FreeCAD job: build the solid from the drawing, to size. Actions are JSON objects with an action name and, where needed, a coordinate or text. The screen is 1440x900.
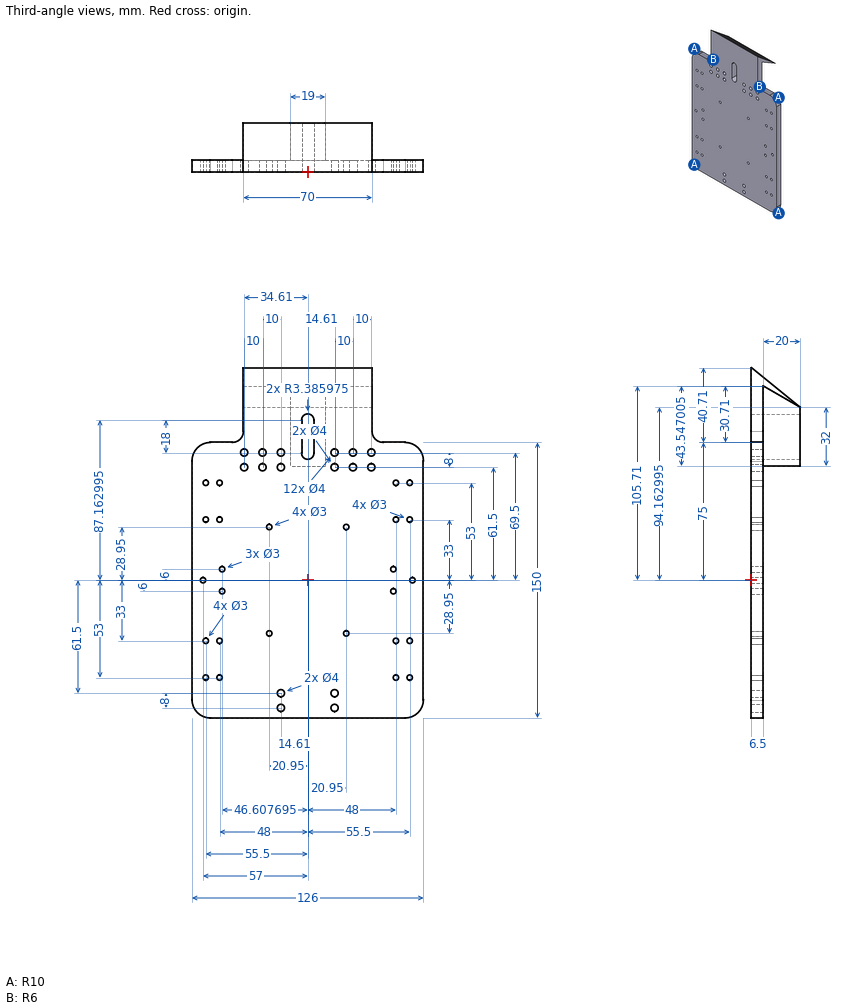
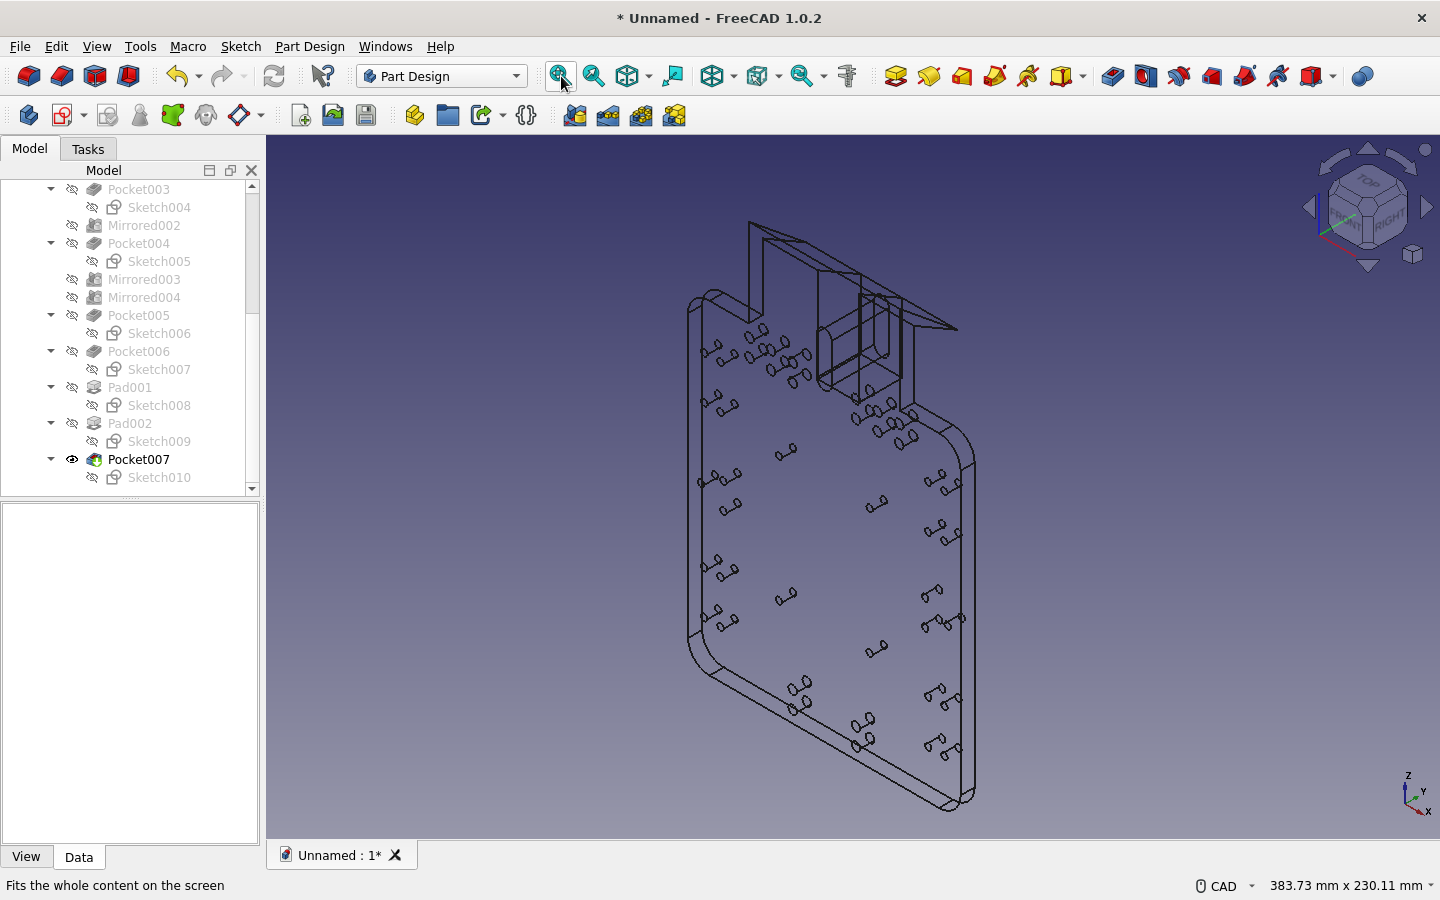
{"action": "left_click", "coordinate": [756, 318]}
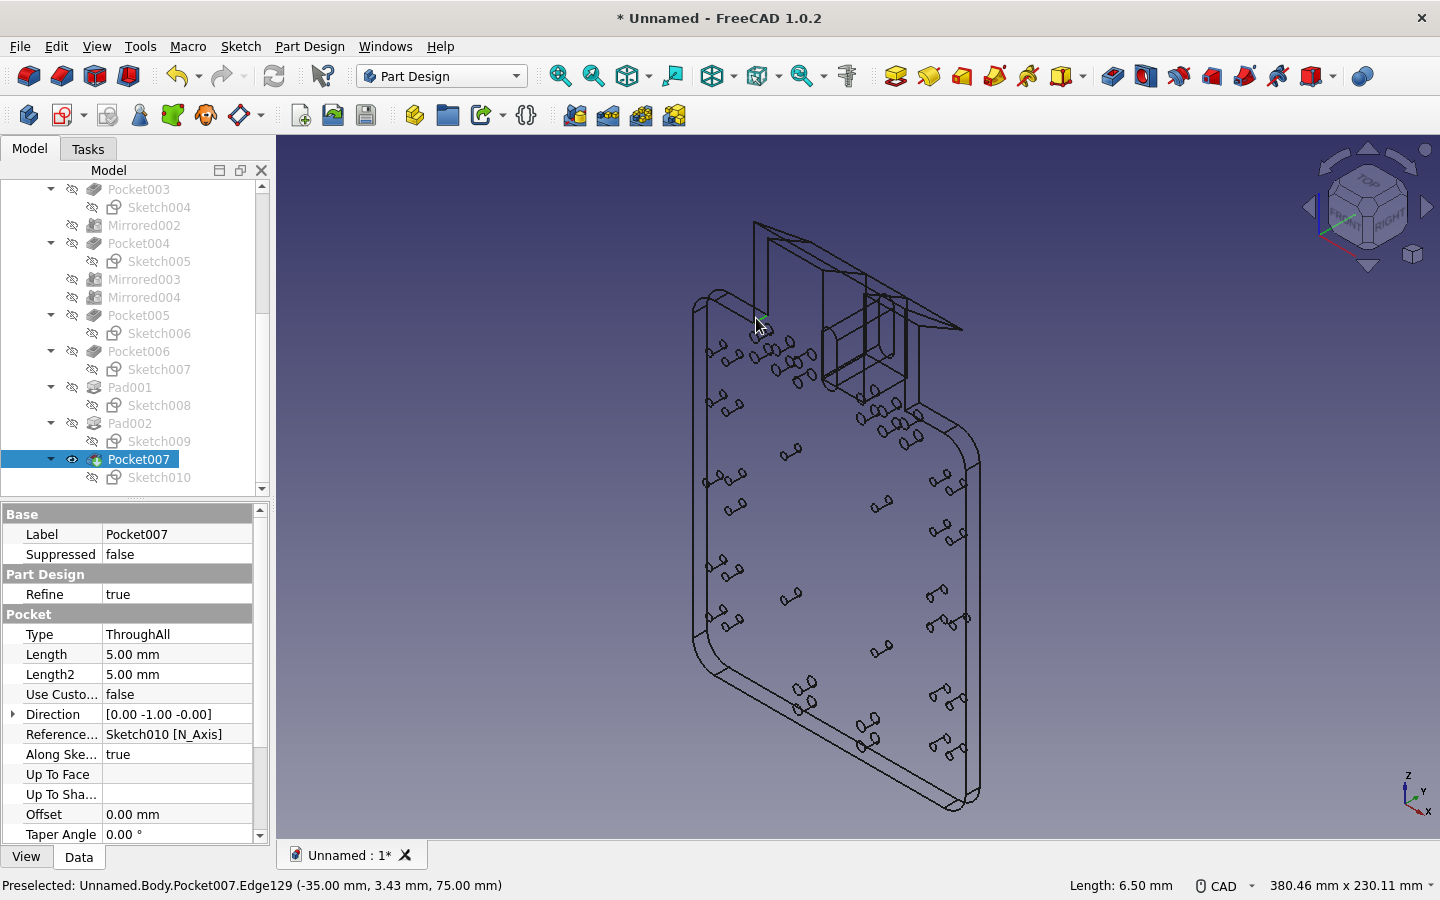
{"action": "left_click", "coordinate": [912, 406], "text": "ctrl"}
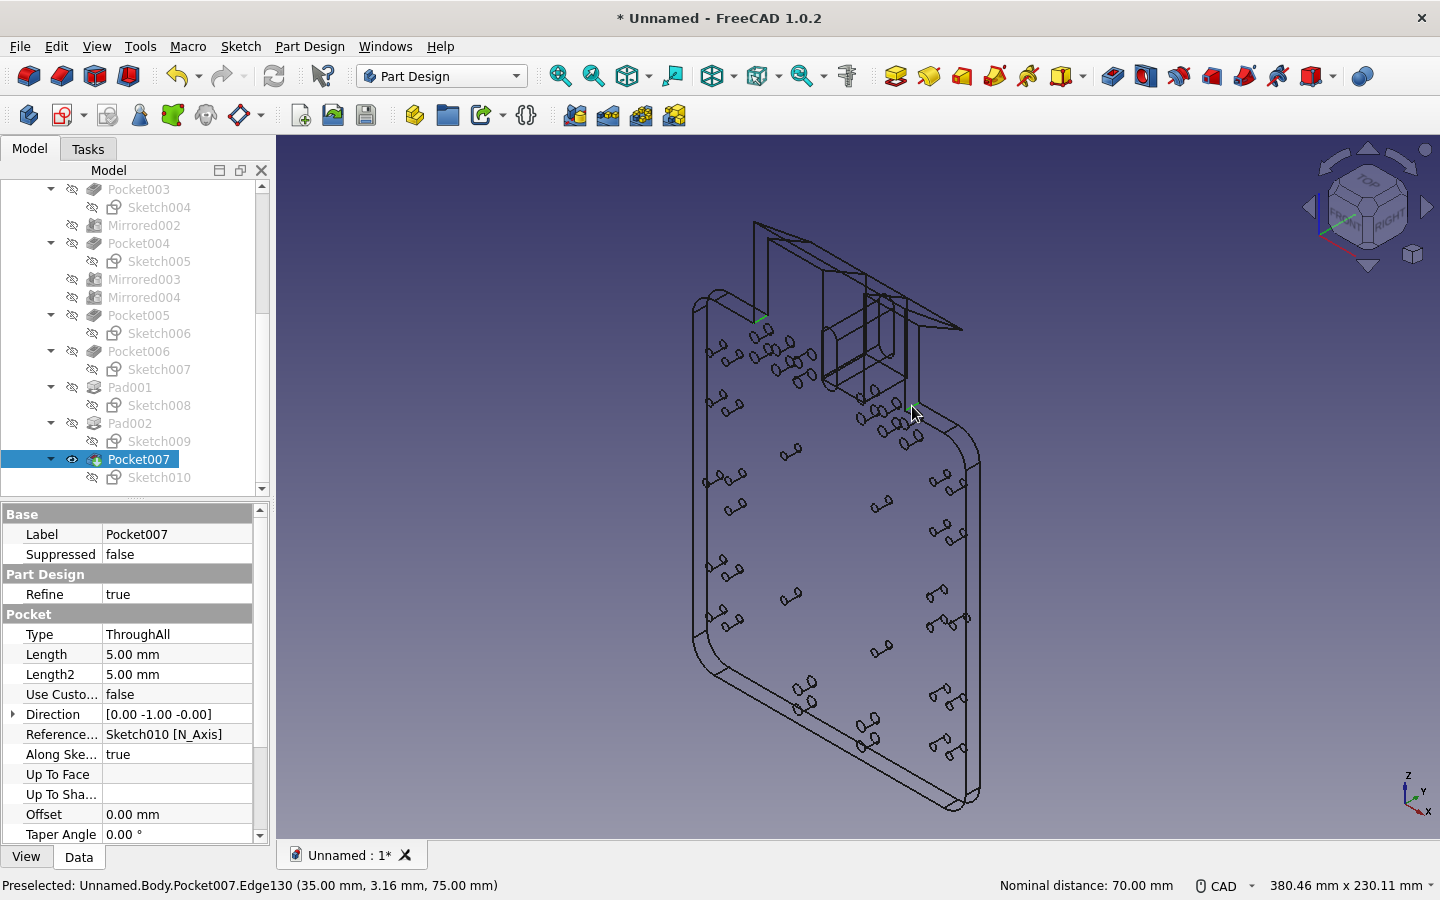
{"action": "key", "text": "v 1"}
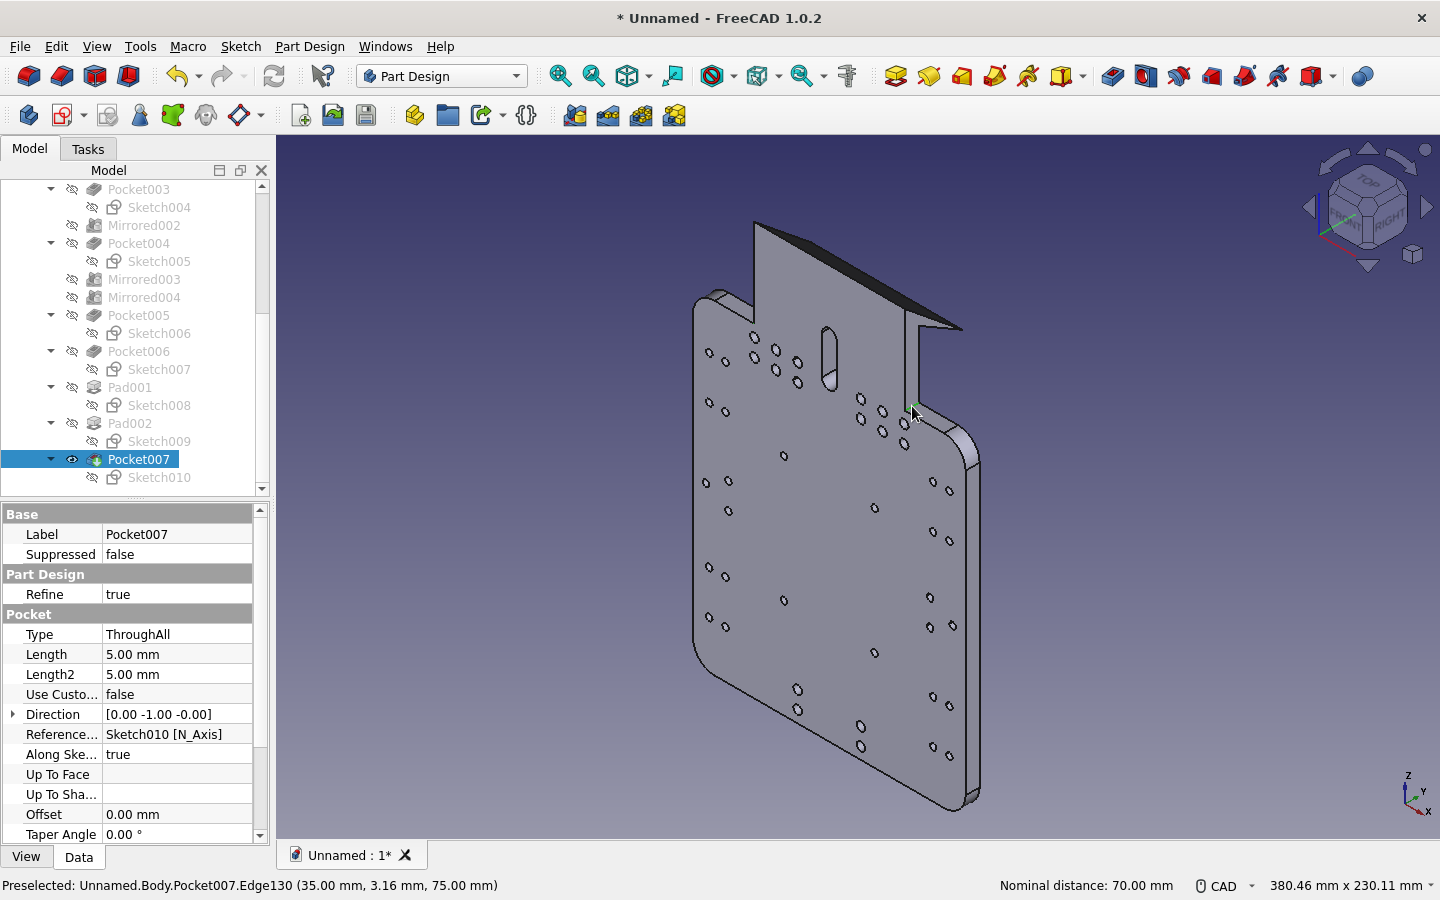
{"action": "left_click", "coordinate": [29, 76]}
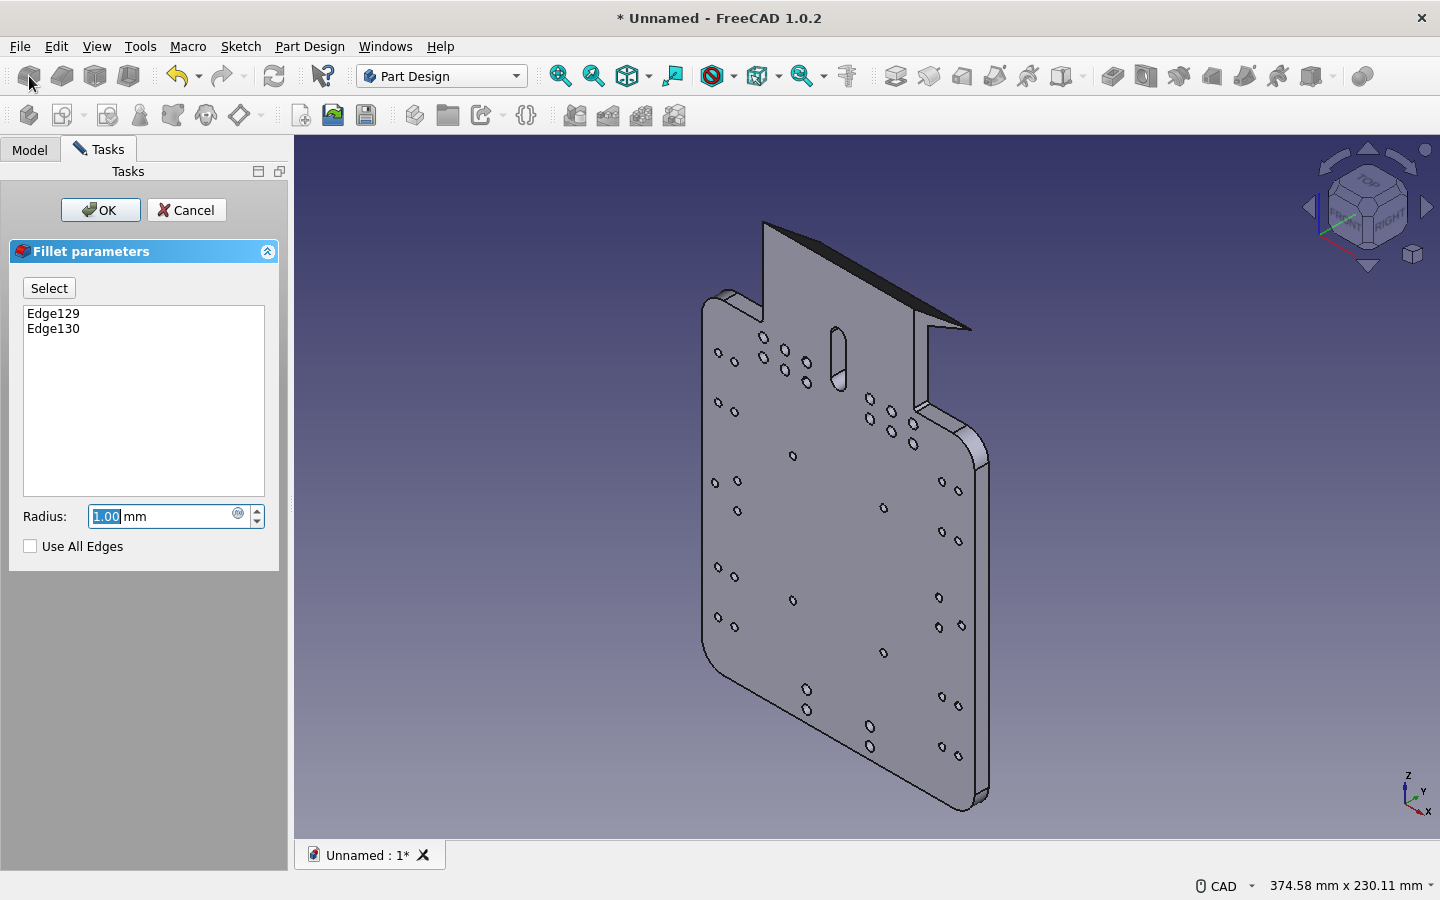
{"action": "type", "text": "6"}
{"action": "key", "text": "Tab"}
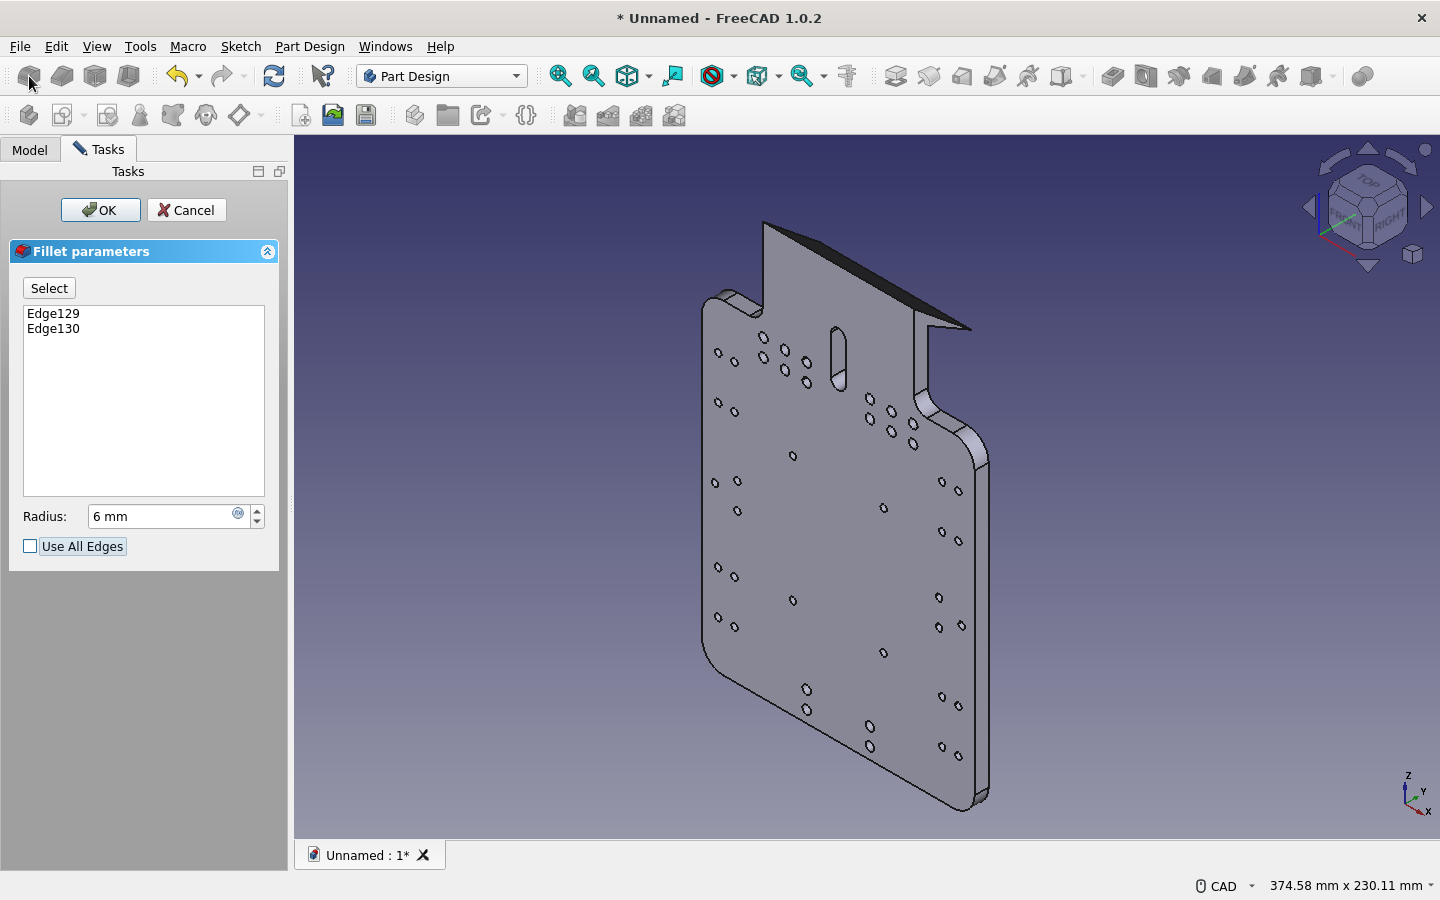
{"action": "left_click", "coordinate": [101, 210]}